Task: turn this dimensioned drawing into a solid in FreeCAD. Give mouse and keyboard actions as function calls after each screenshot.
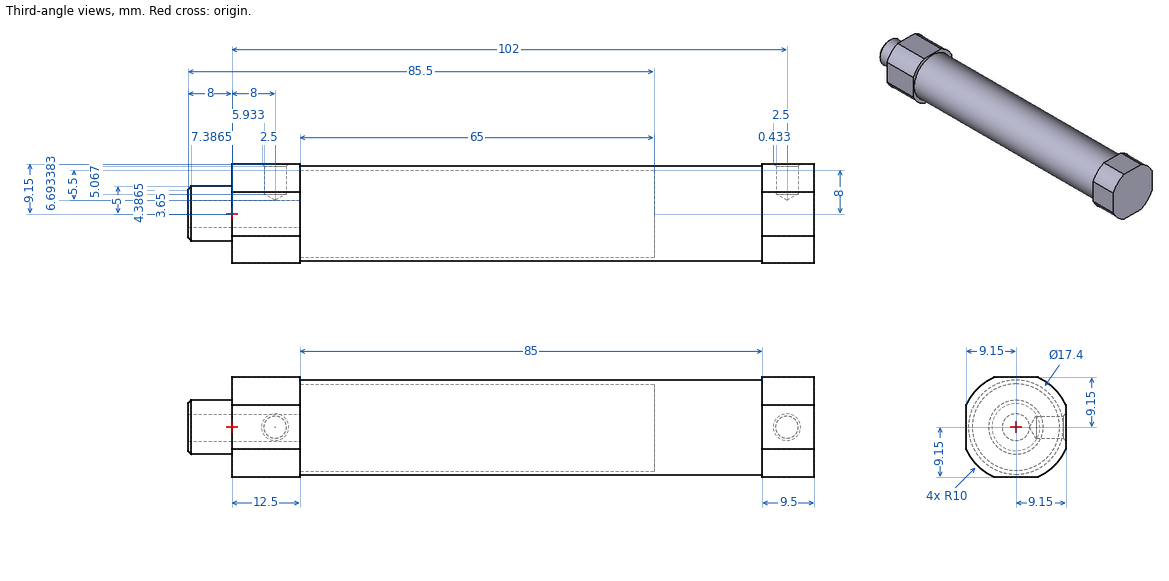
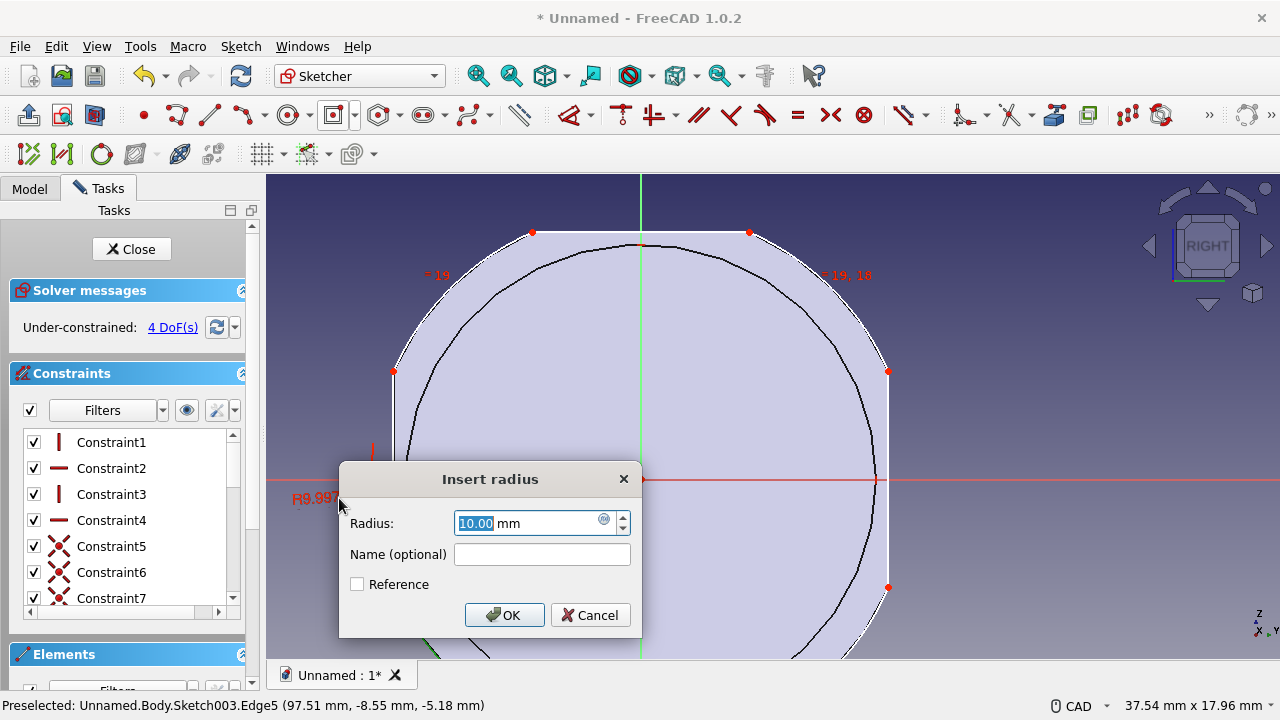
text(10)
key(Return)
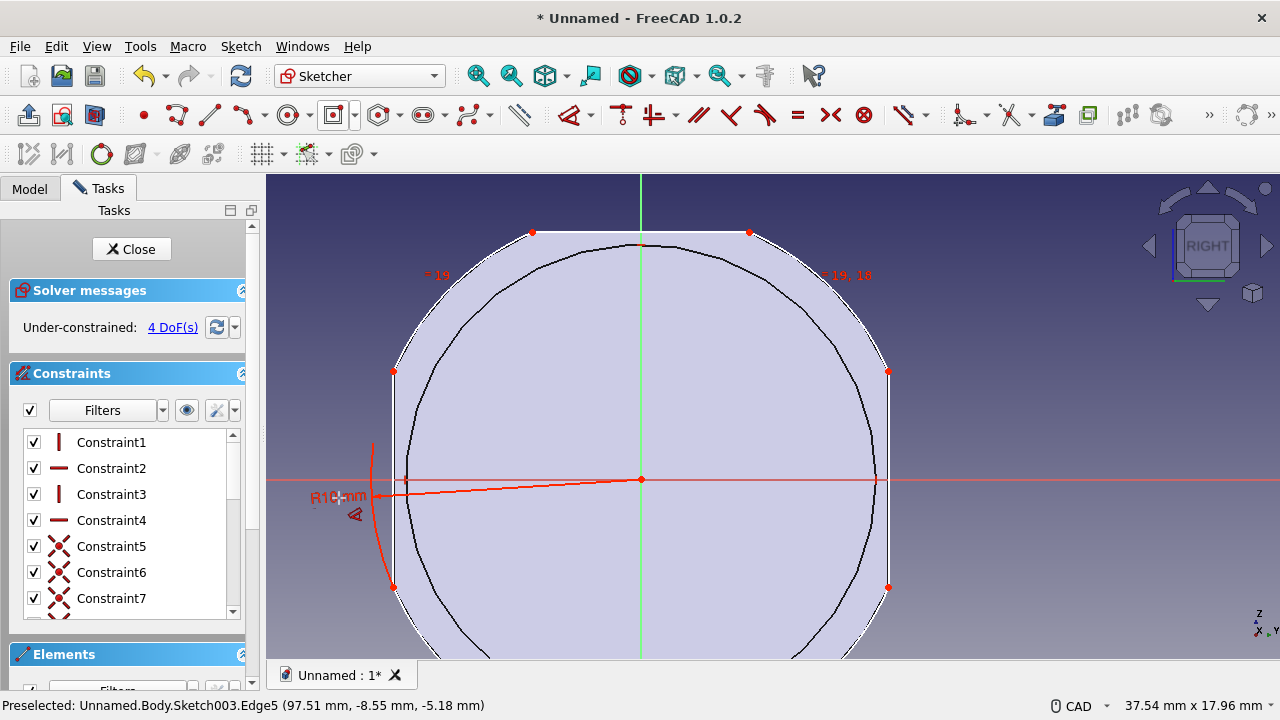
click(393, 372)
click(517, 338)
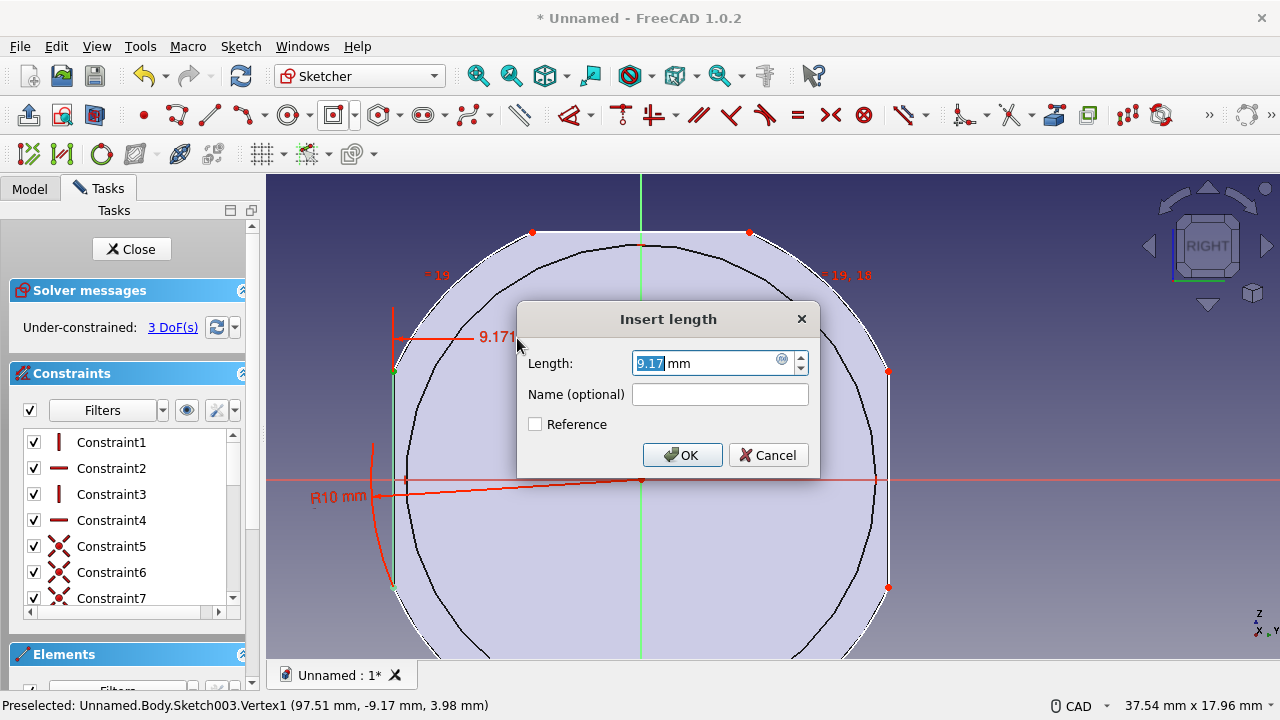
text(9.15)
key(Return)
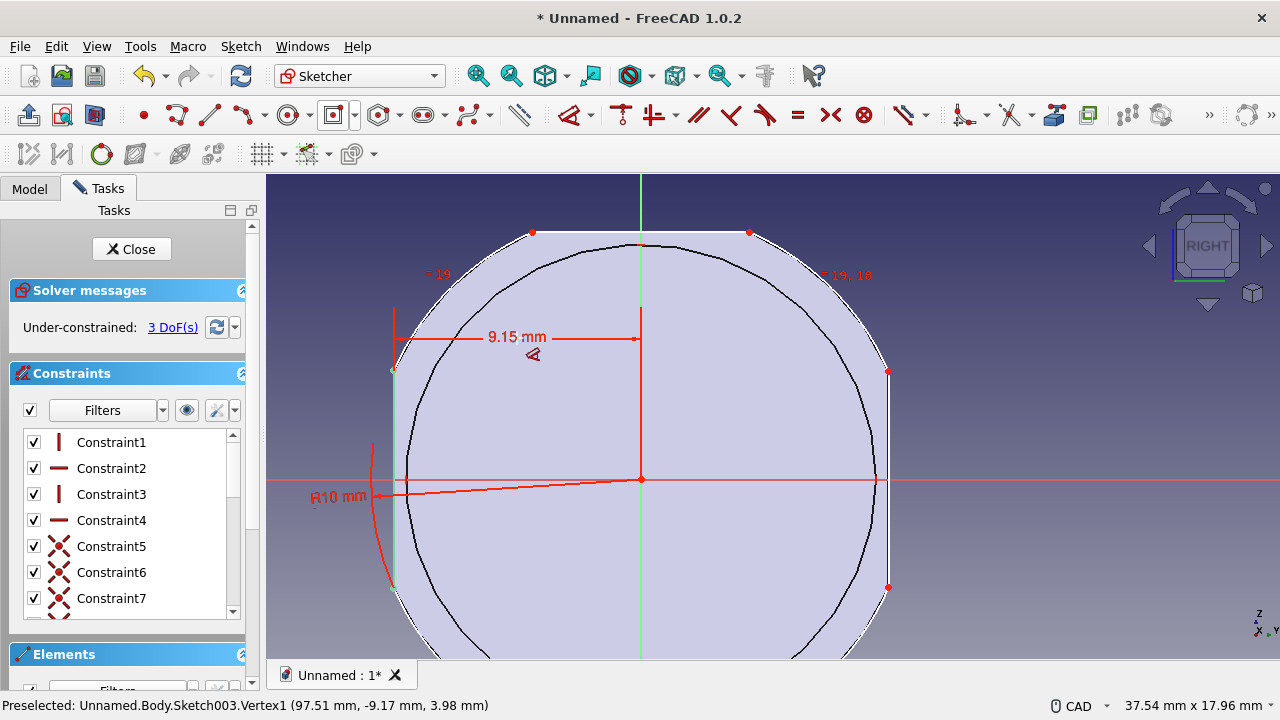
scroll(833, 288, down, 2)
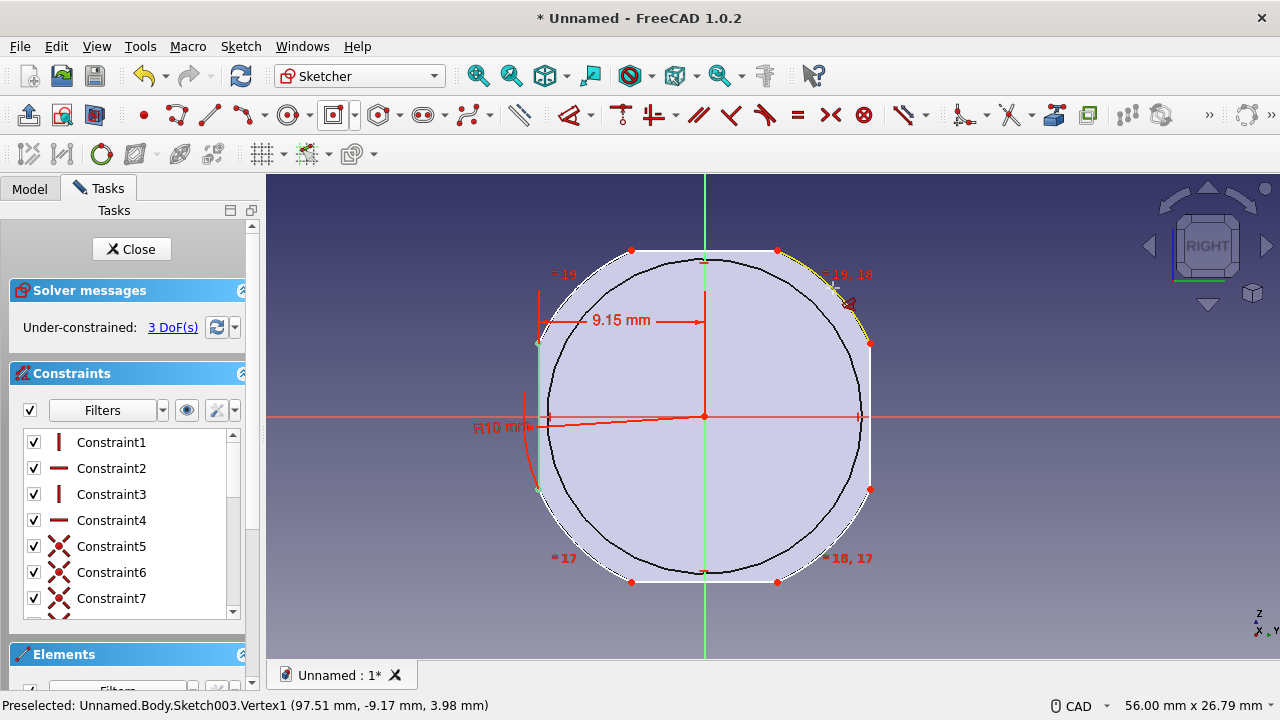
click(632, 582)
click(598, 499)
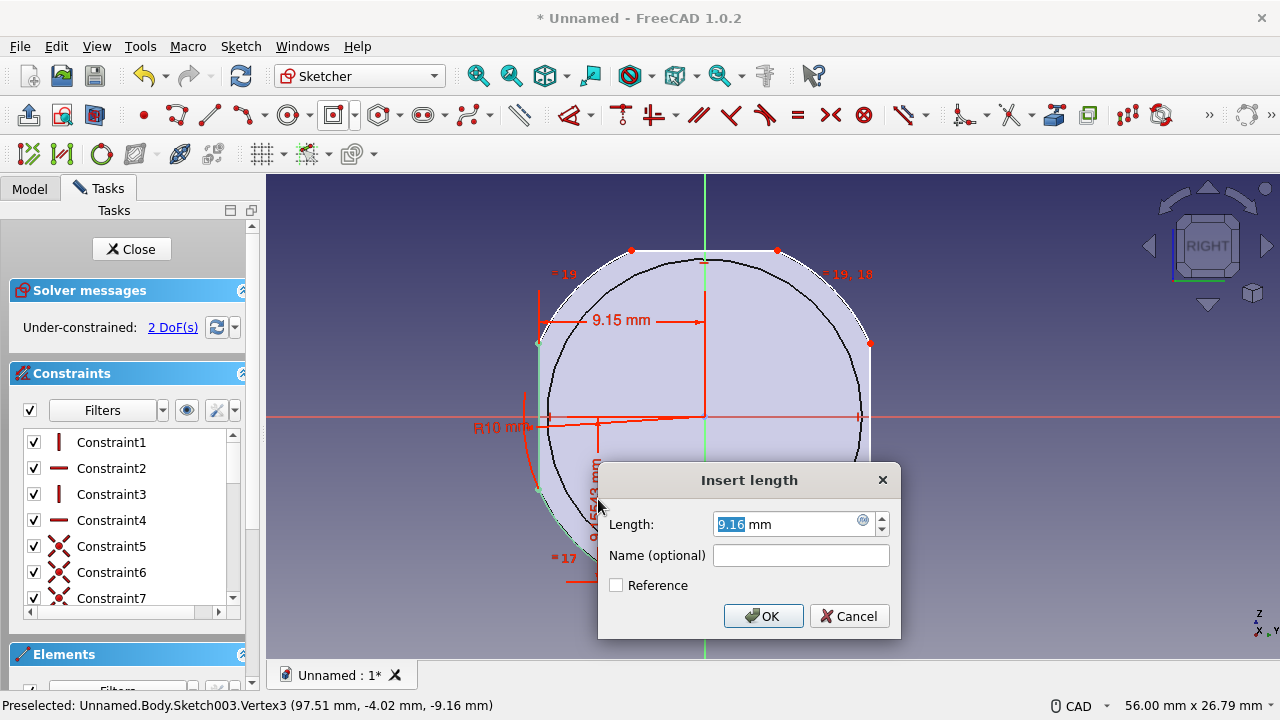
text(9.15)
key(Return)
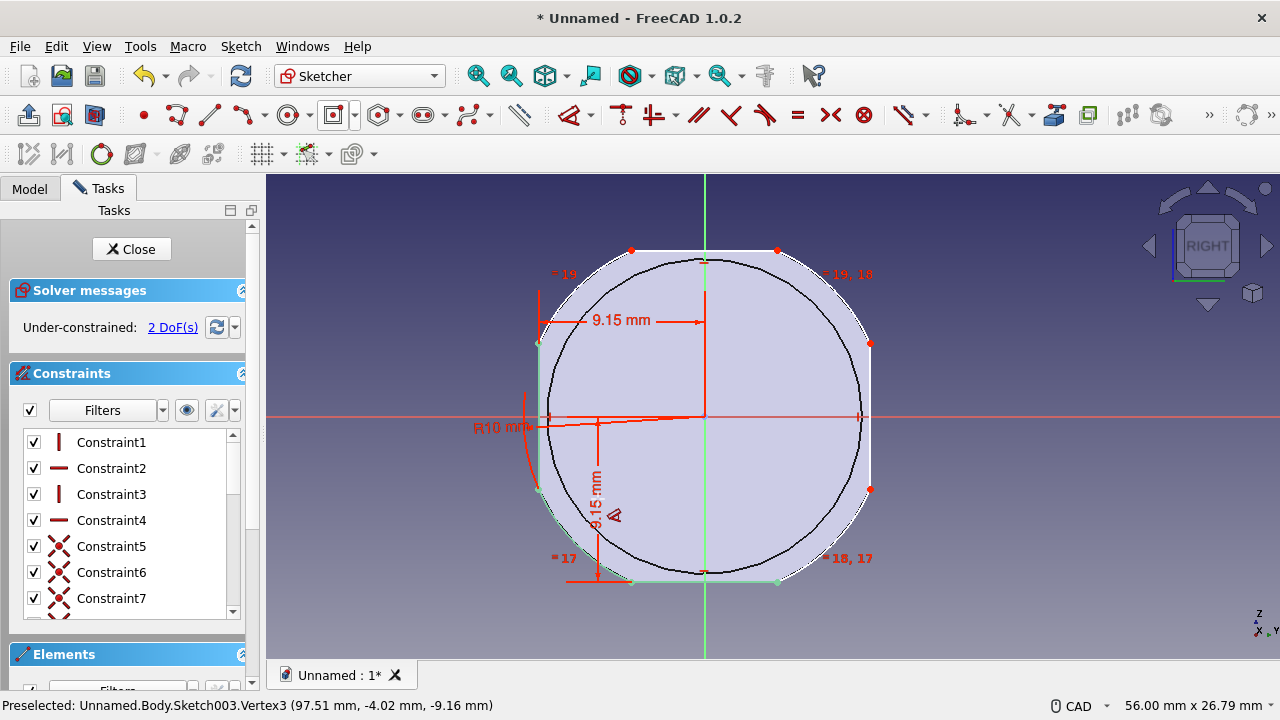
click(870, 489)
click(787, 523)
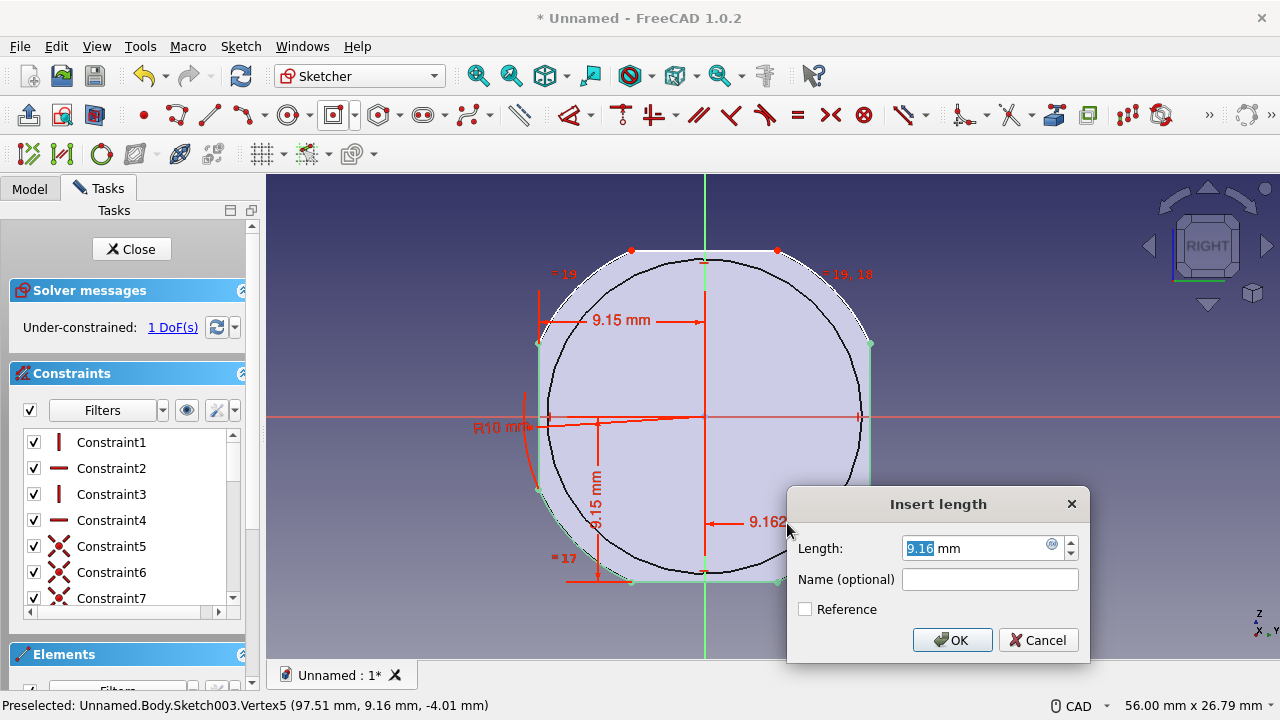
text(9.15)
key(Return)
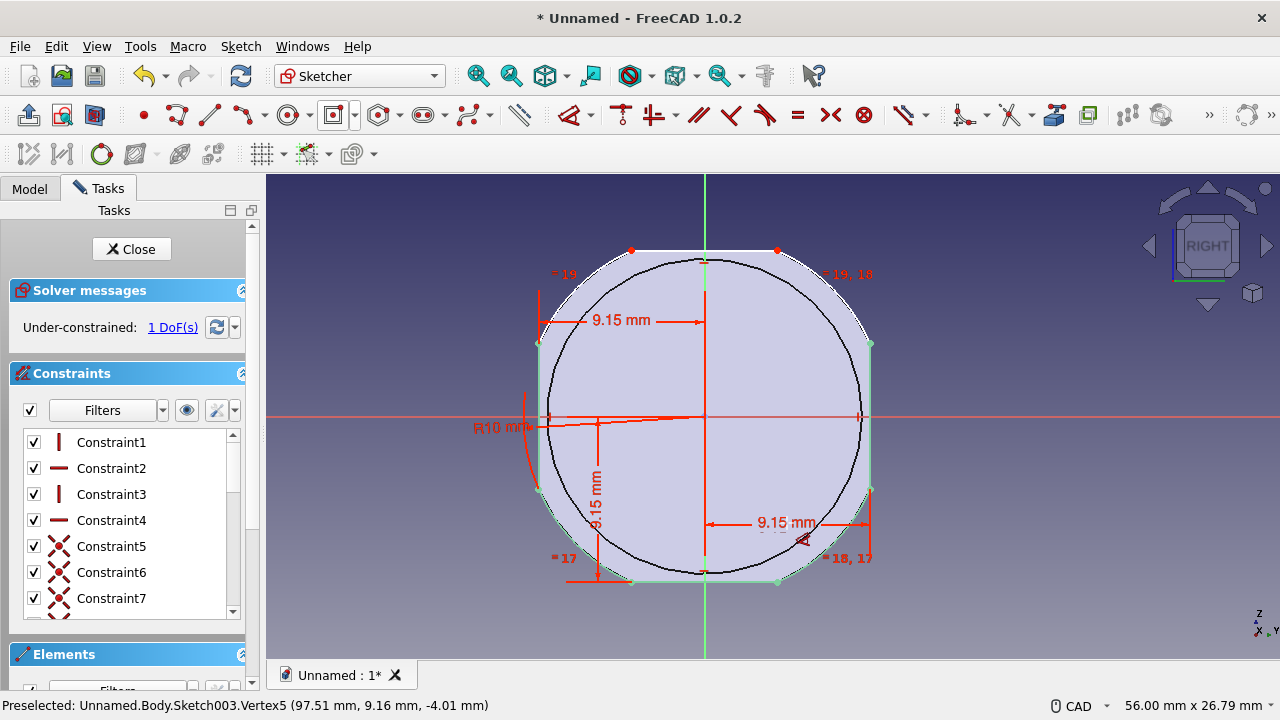
click(777, 251)
click(811, 334)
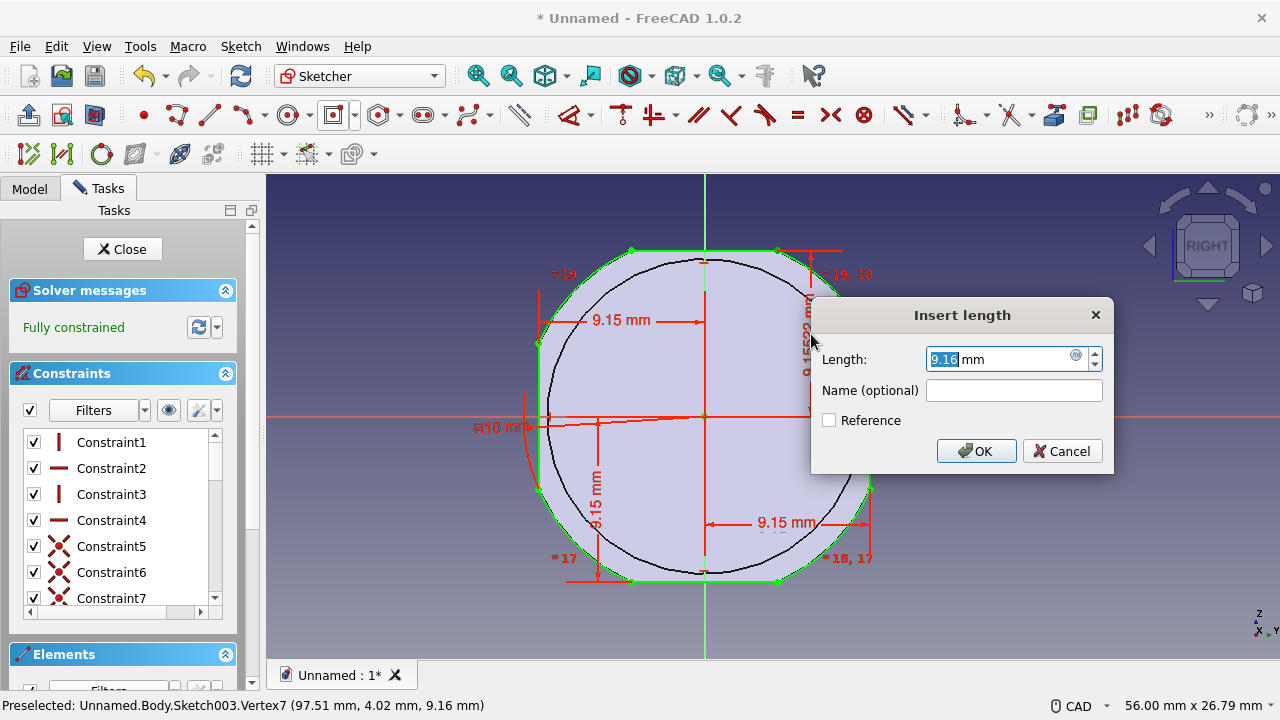
text(9.15)
key(Return)
key(Escape)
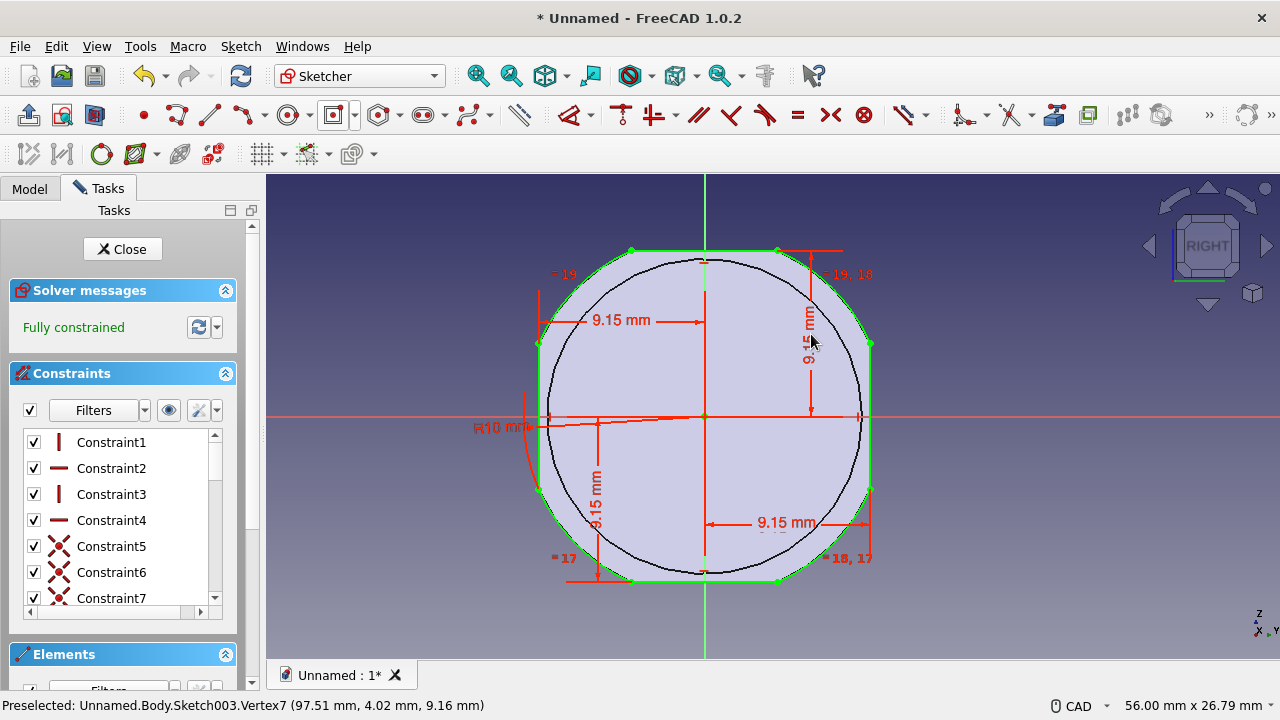
click(123, 249)